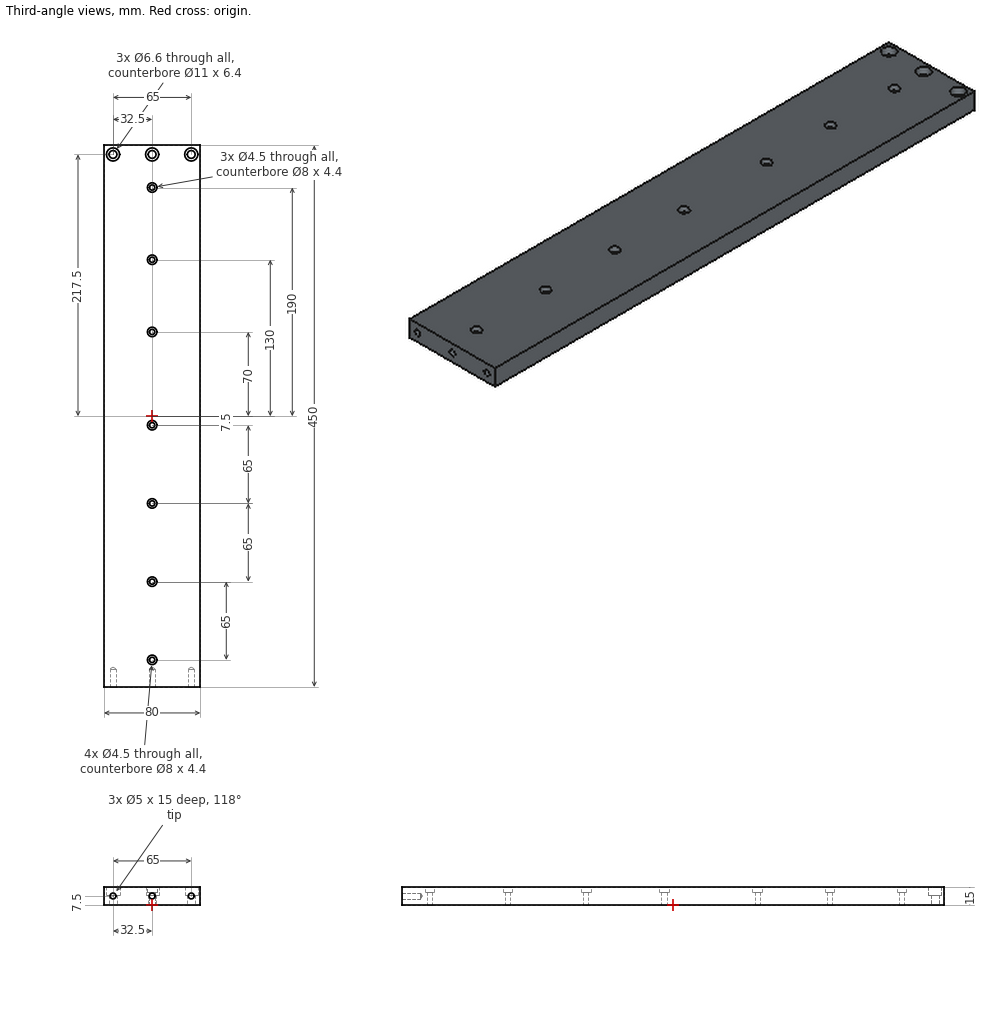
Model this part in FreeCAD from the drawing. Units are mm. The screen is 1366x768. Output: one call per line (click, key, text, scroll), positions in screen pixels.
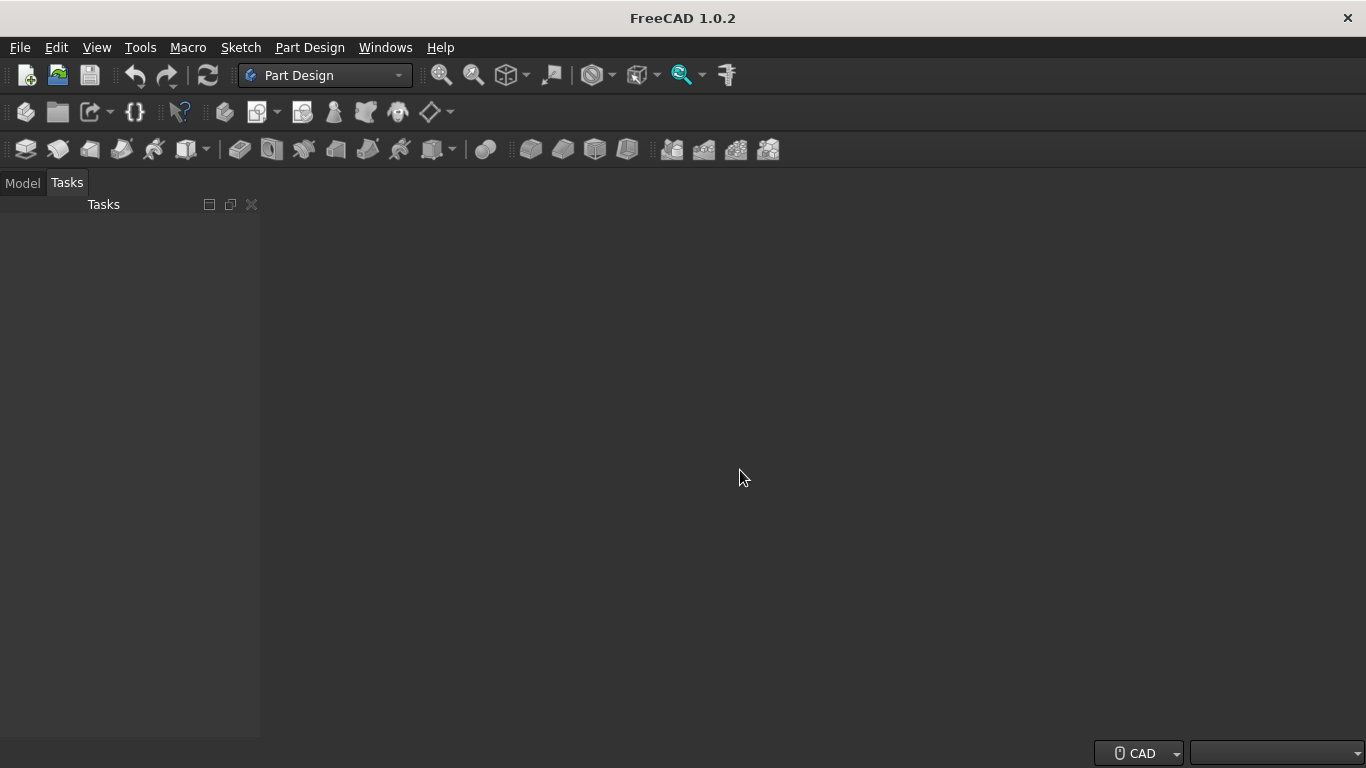
click(26, 76)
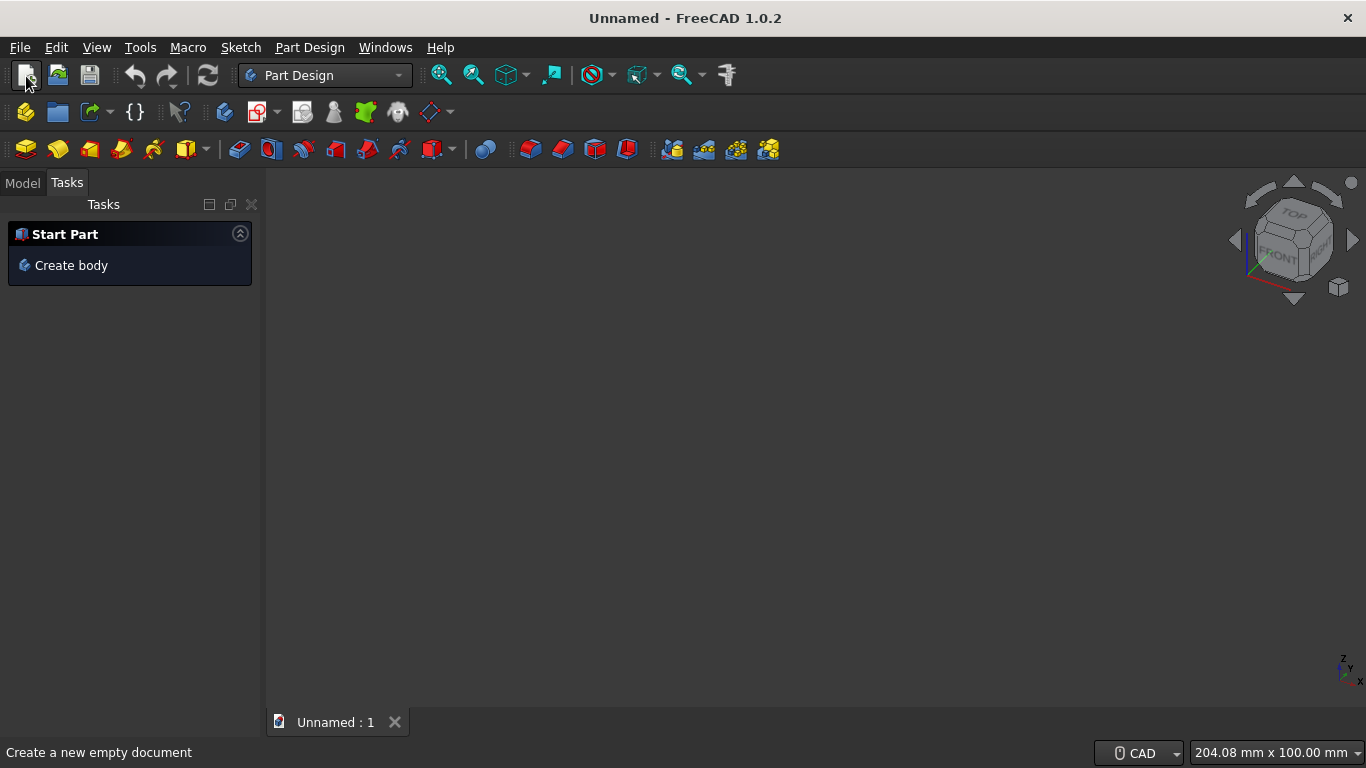
click(258, 112)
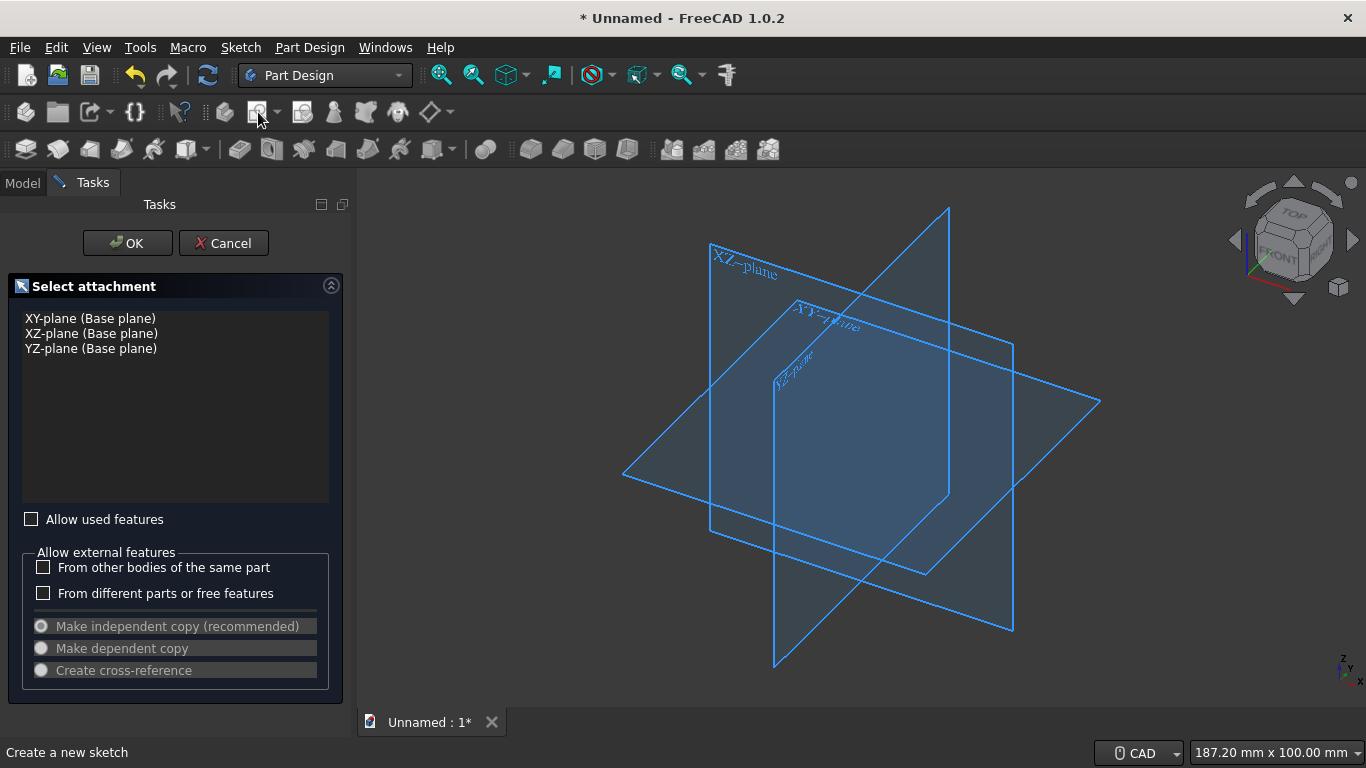
click(82, 318)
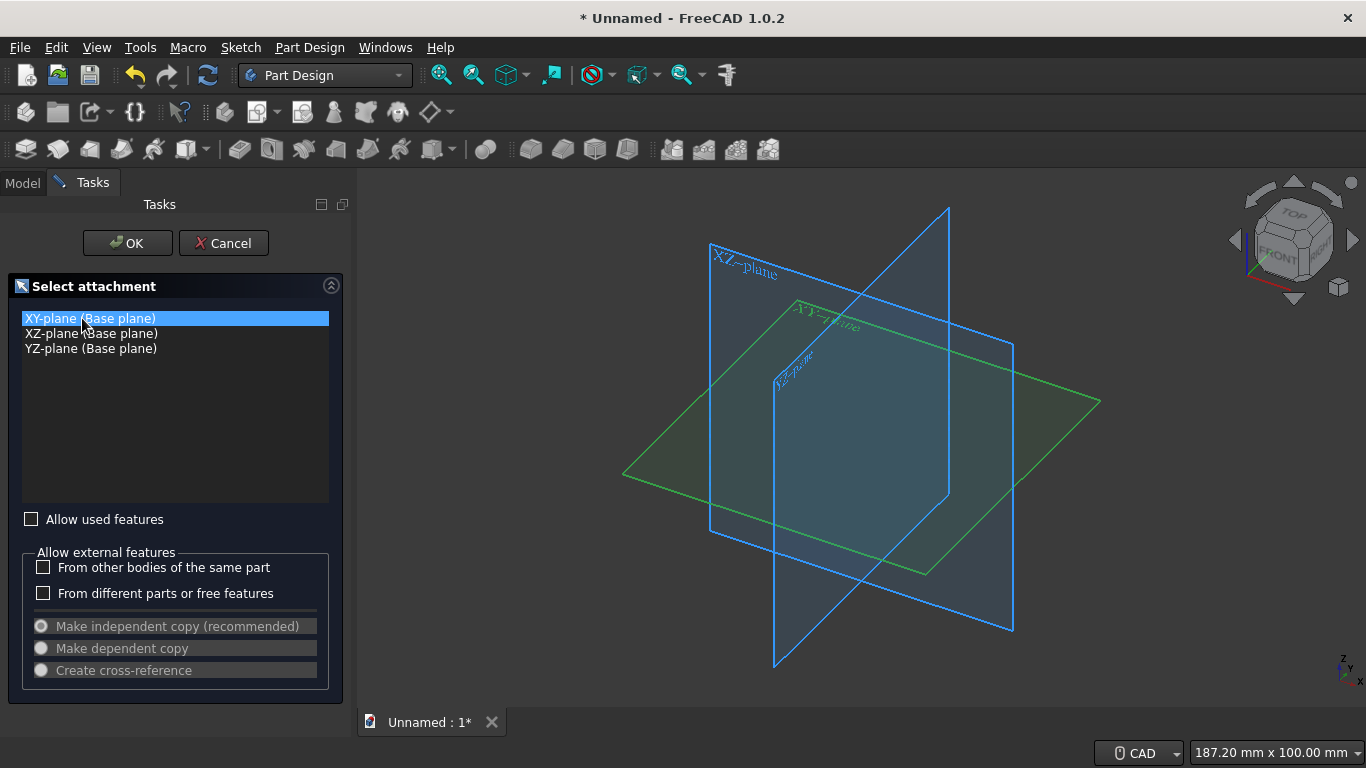
click(128, 243)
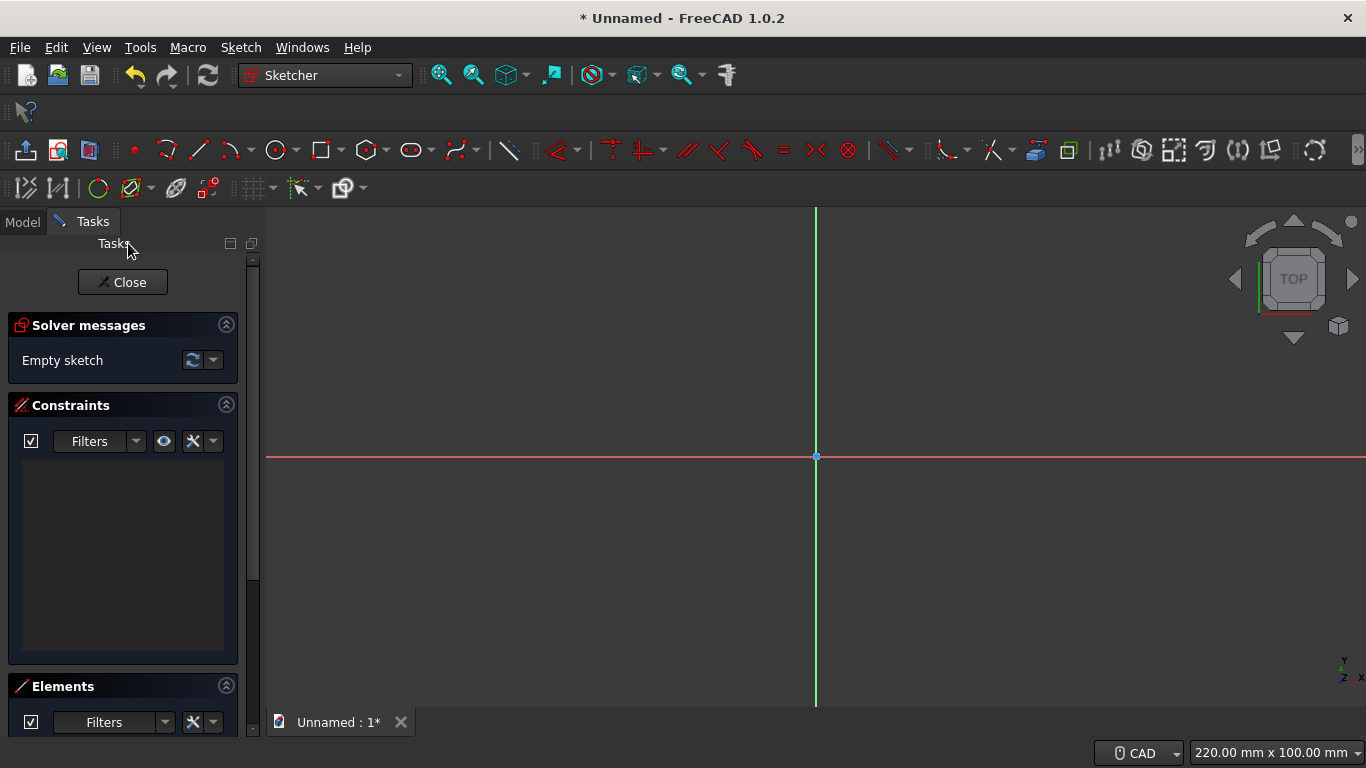
scroll(737, 457, down, 10)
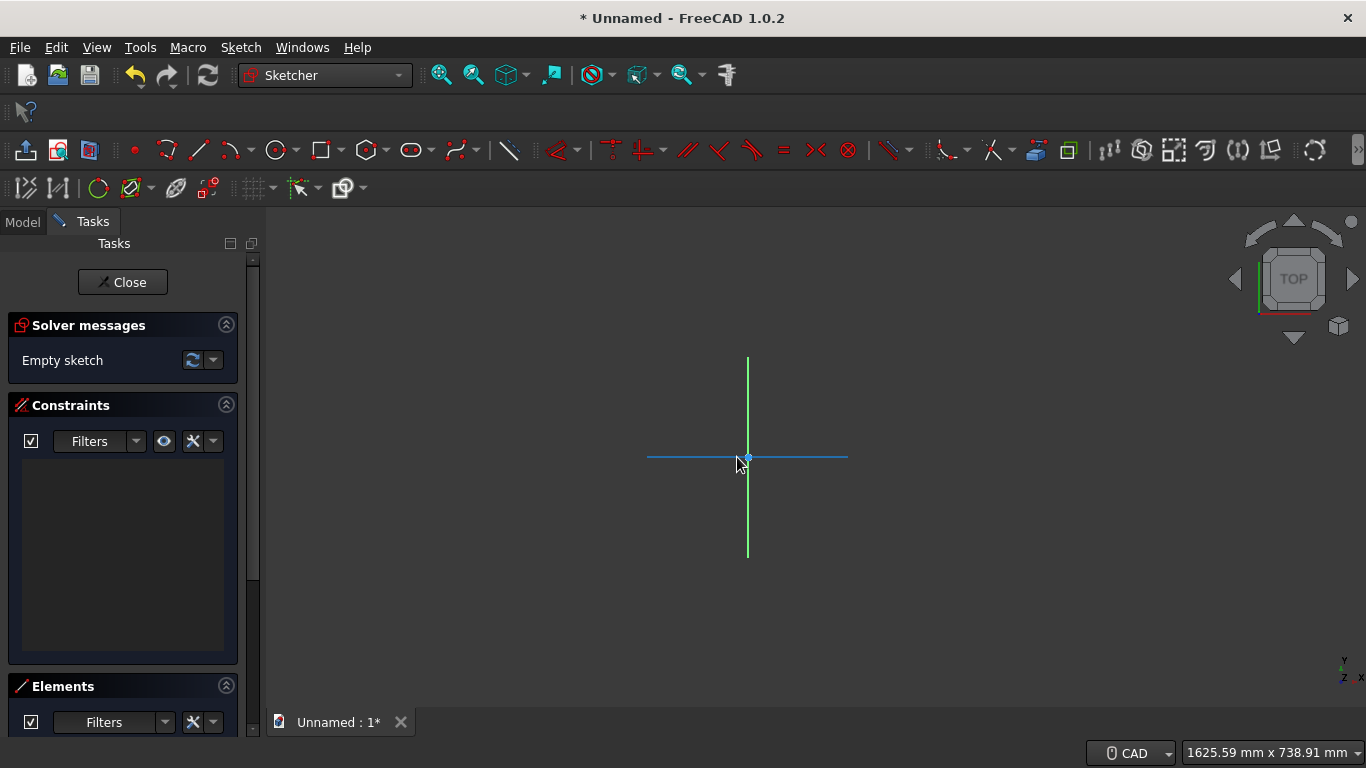
key(g)
key(v)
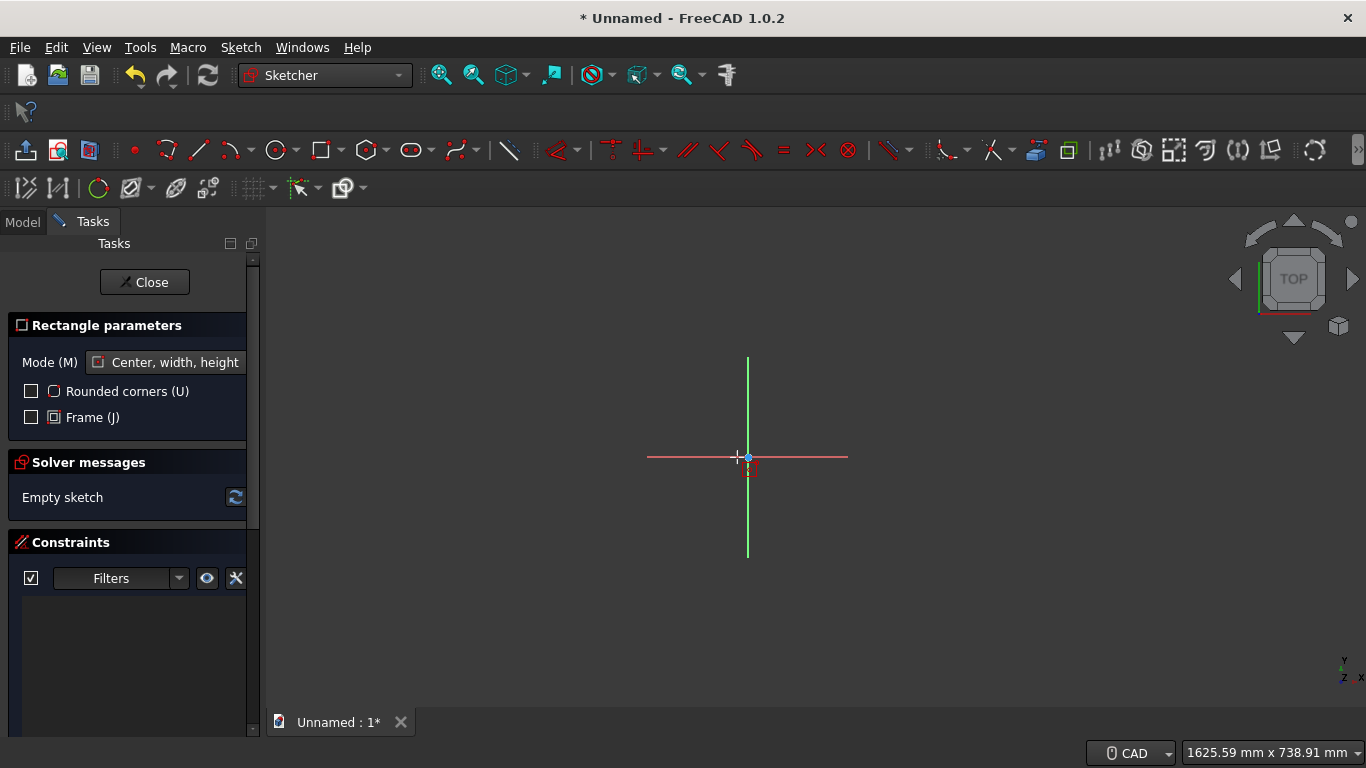
click(748, 457)
move(775, 305)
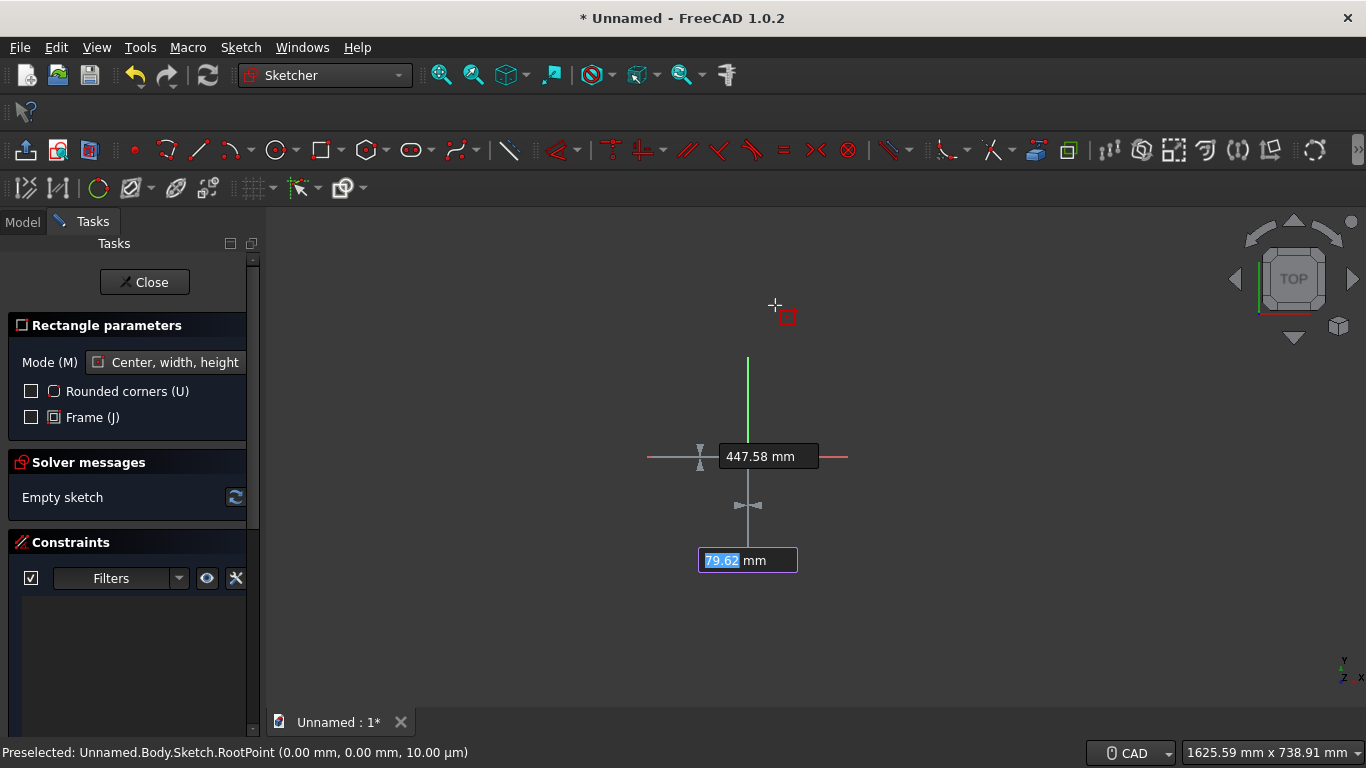
text(80)
key(Tab)
text(450)
key(Return)
key(Escape)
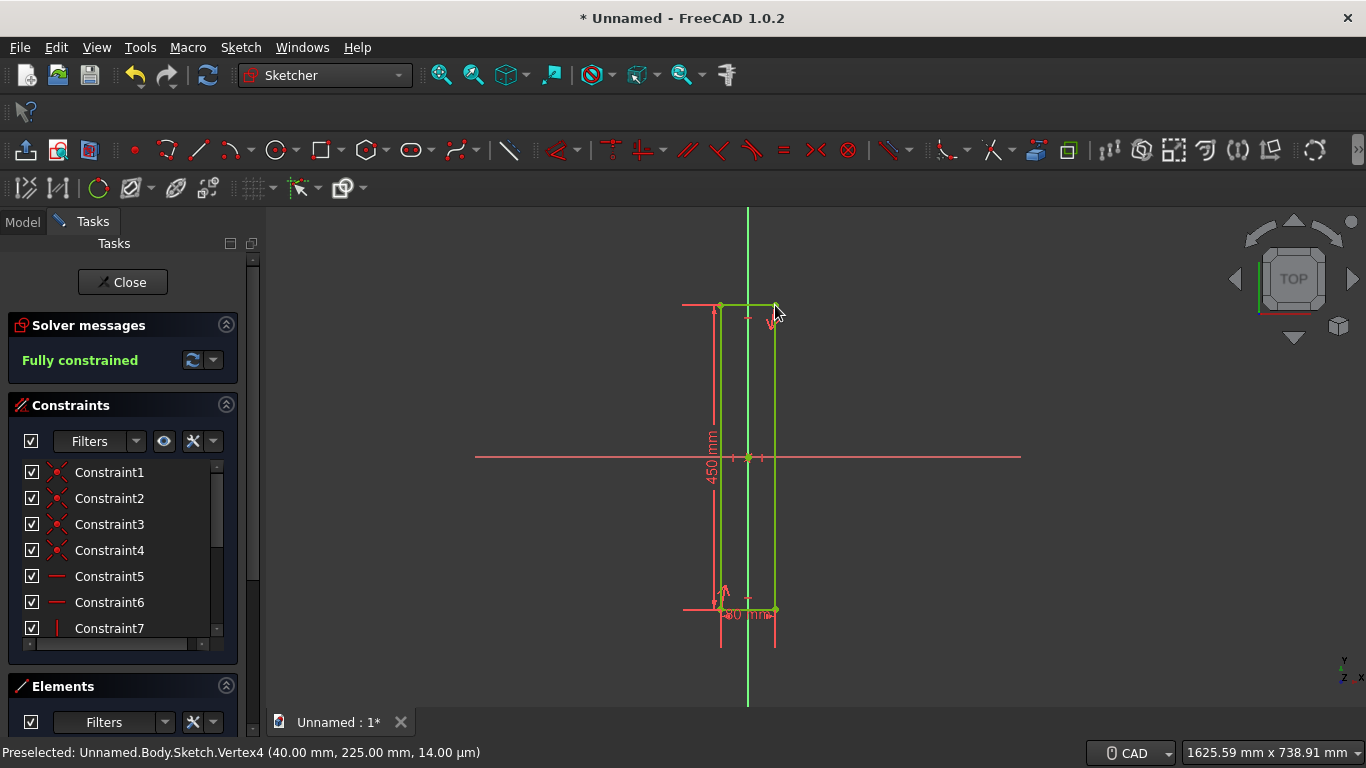
click(123, 282)